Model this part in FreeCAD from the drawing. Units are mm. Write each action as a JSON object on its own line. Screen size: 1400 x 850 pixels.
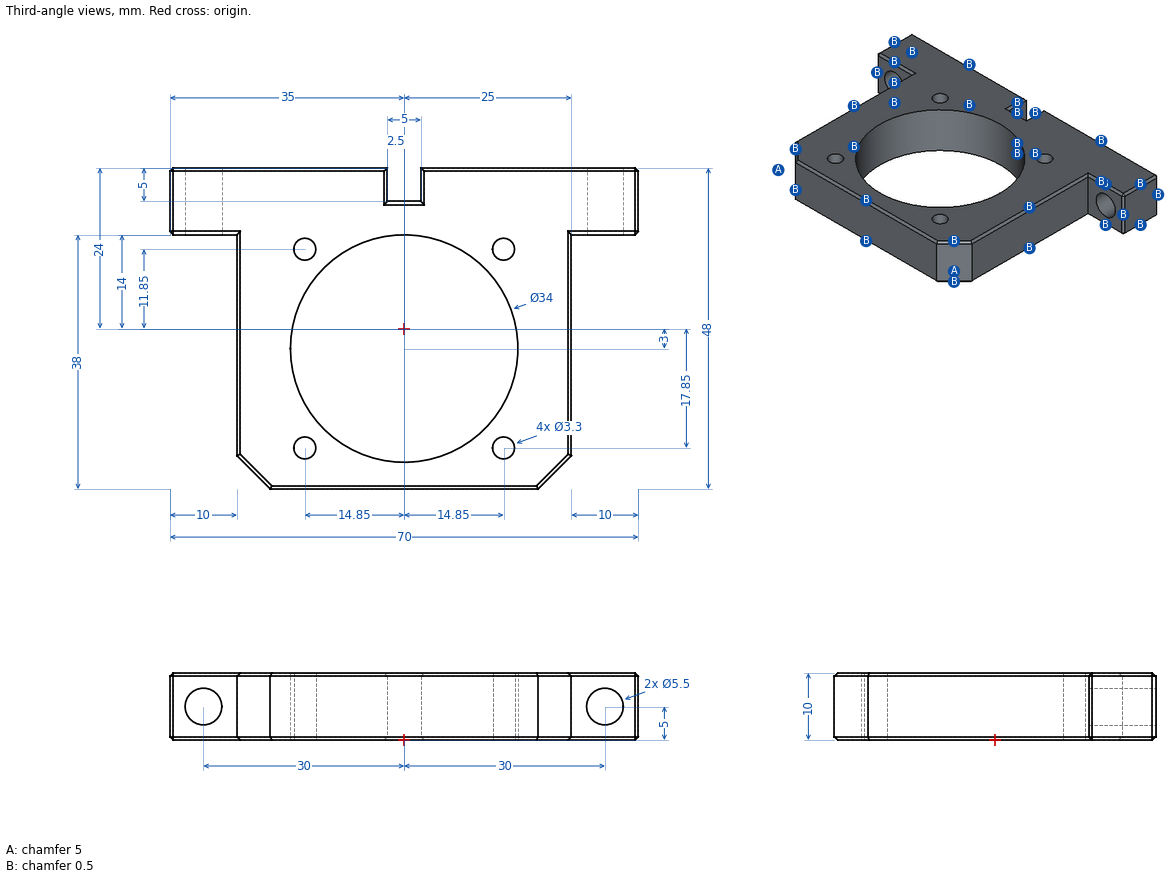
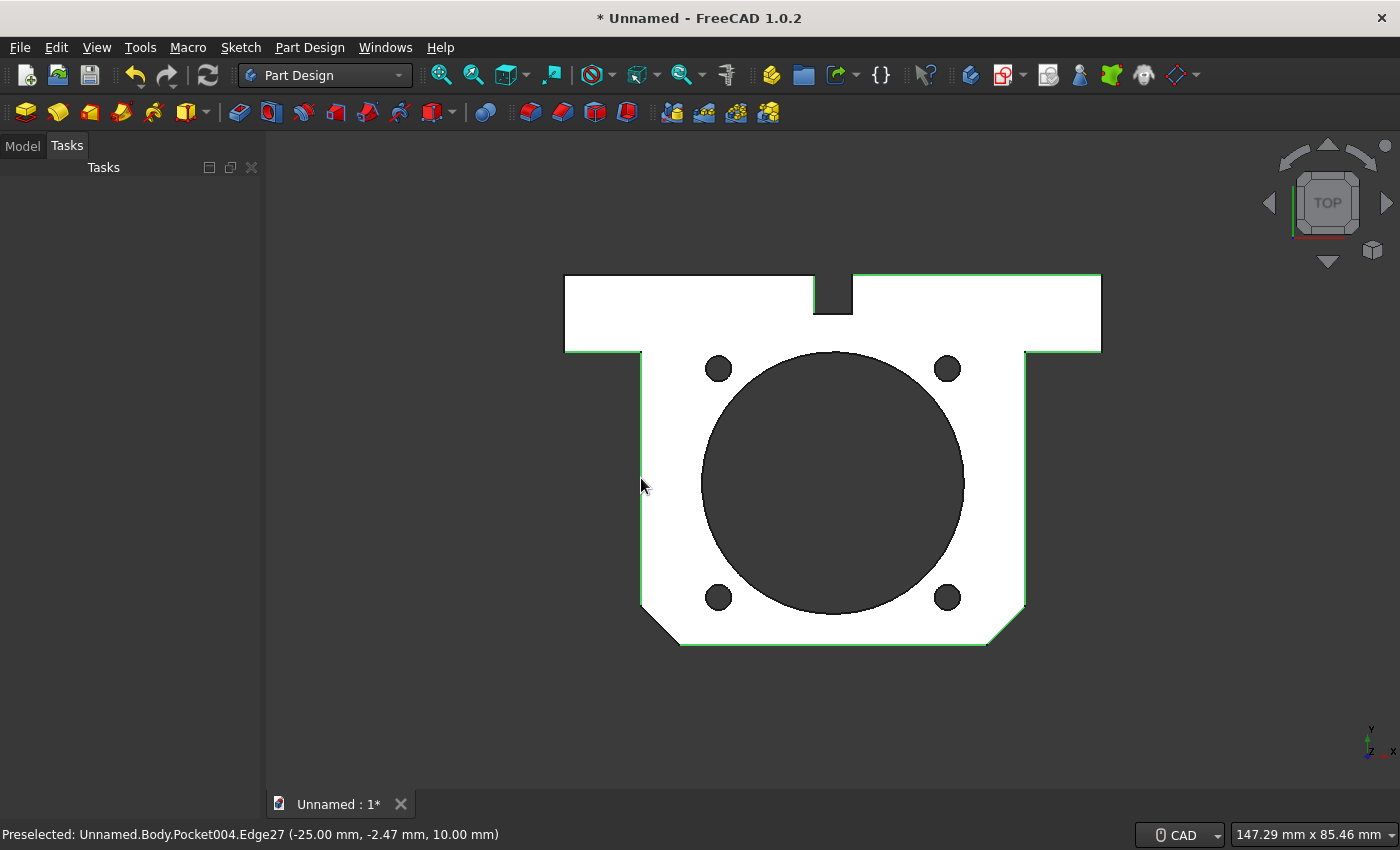
{"action": "left_click", "coordinate": [660, 625], "text": "ctrl"}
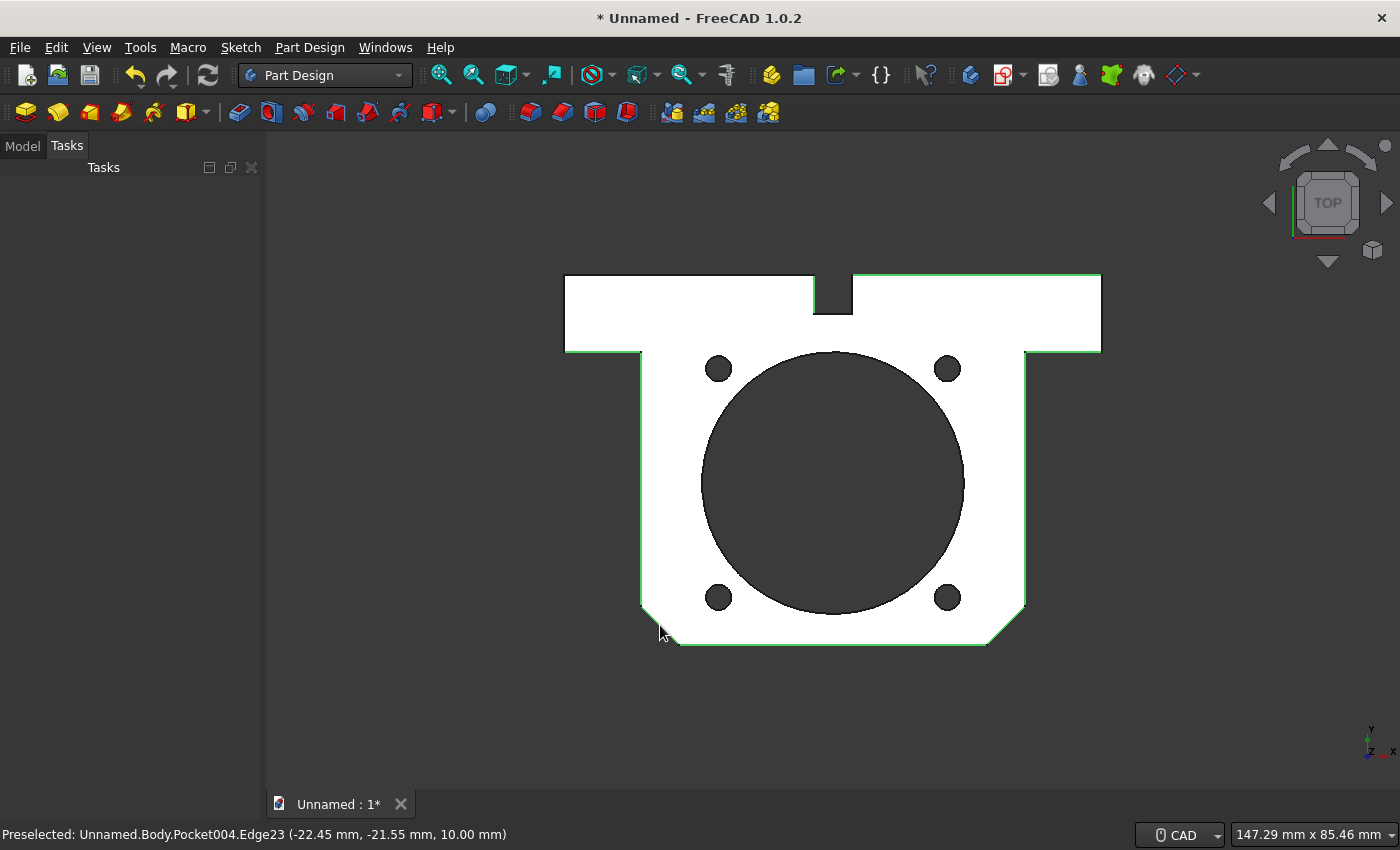
{"action": "left_click", "coordinate": [689, 274], "text": "ctrl"}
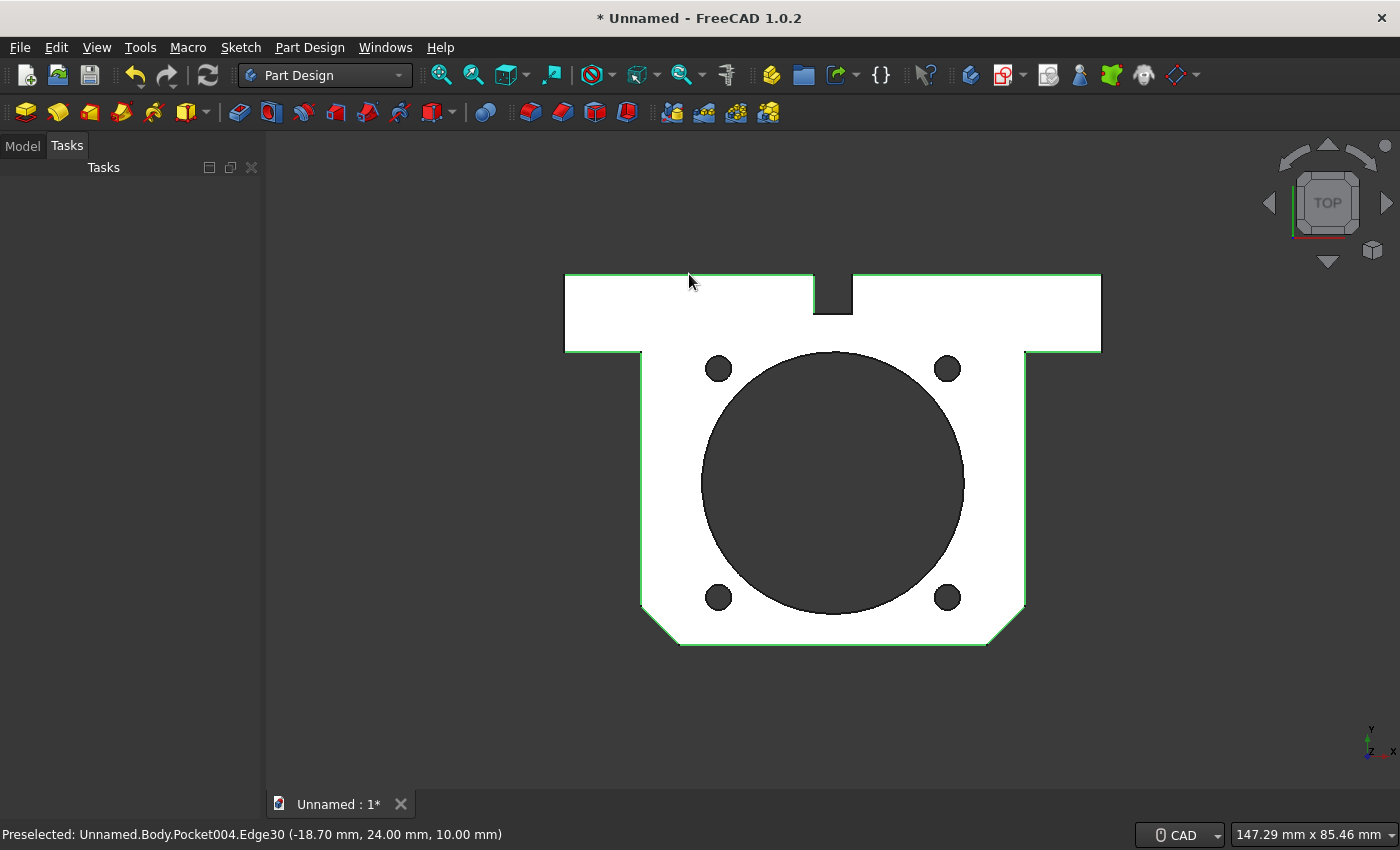
{"action": "left_click", "coordinate": [833, 313], "text": "ctrl"}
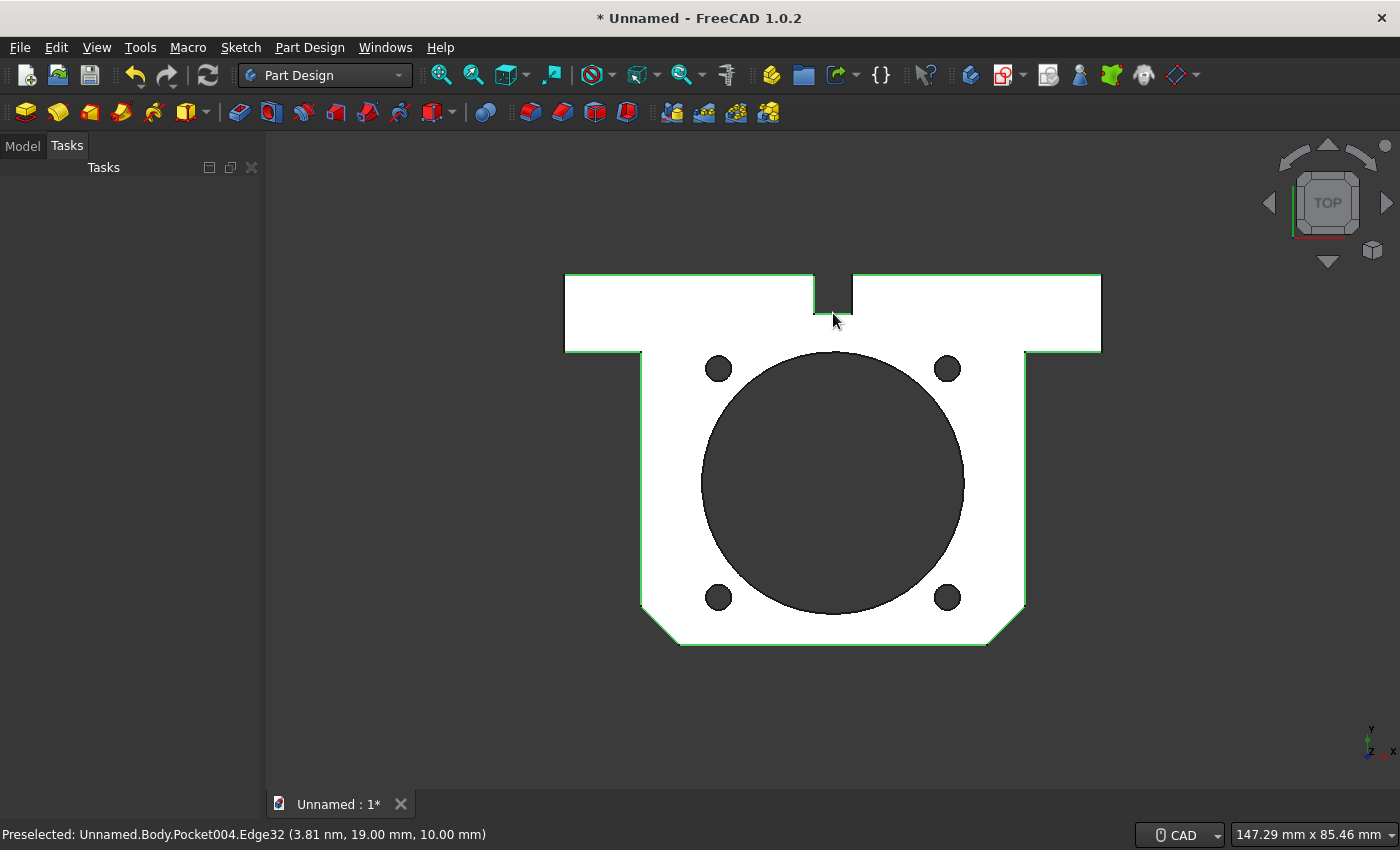
{"action": "left_click", "coordinate": [852, 293], "text": "ctrl"}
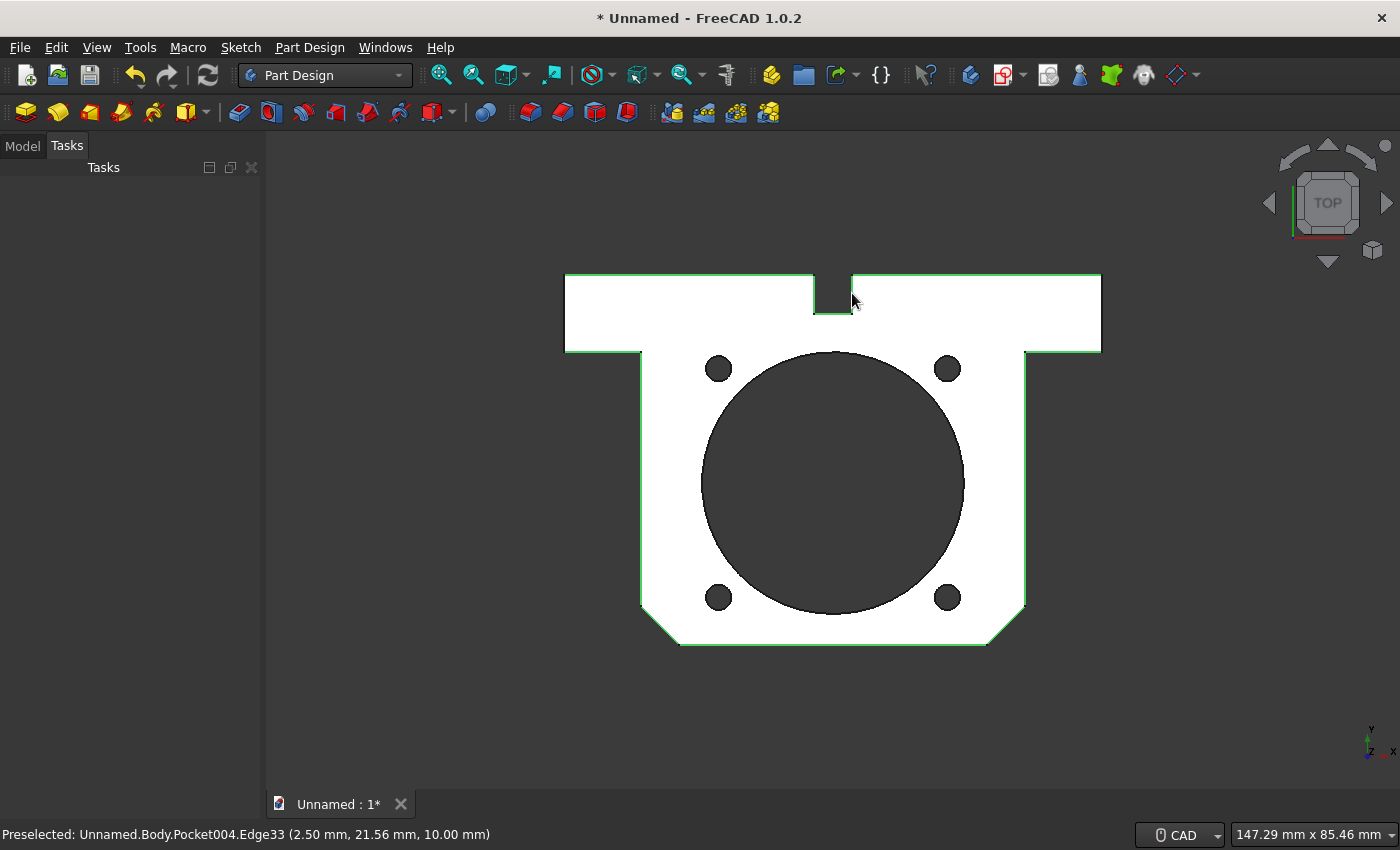
{"action": "key", "text": "0"}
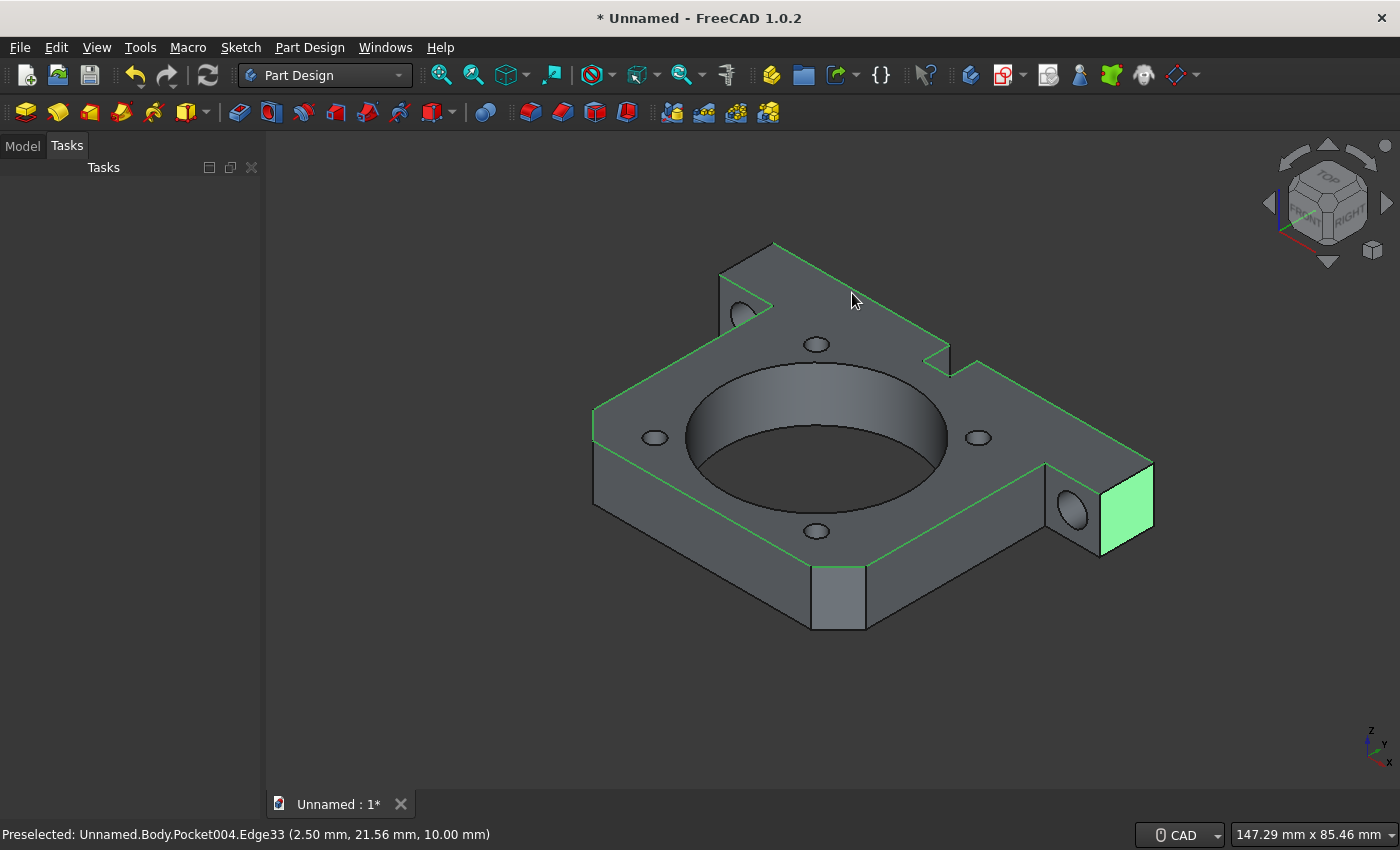
{"action": "key", "text": "1"}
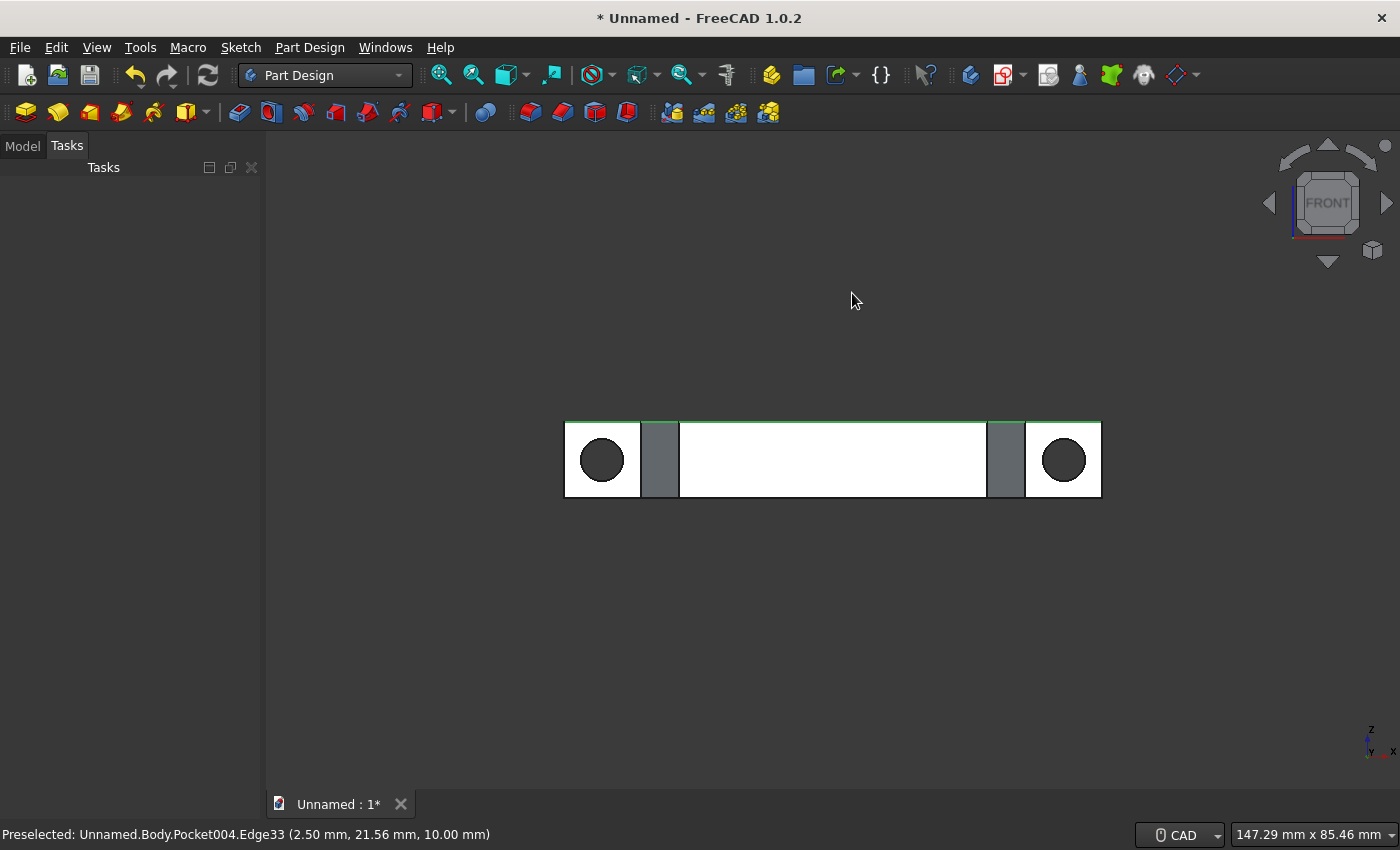
{"action": "left_click", "coordinate": [602, 497], "text": "ctrl"}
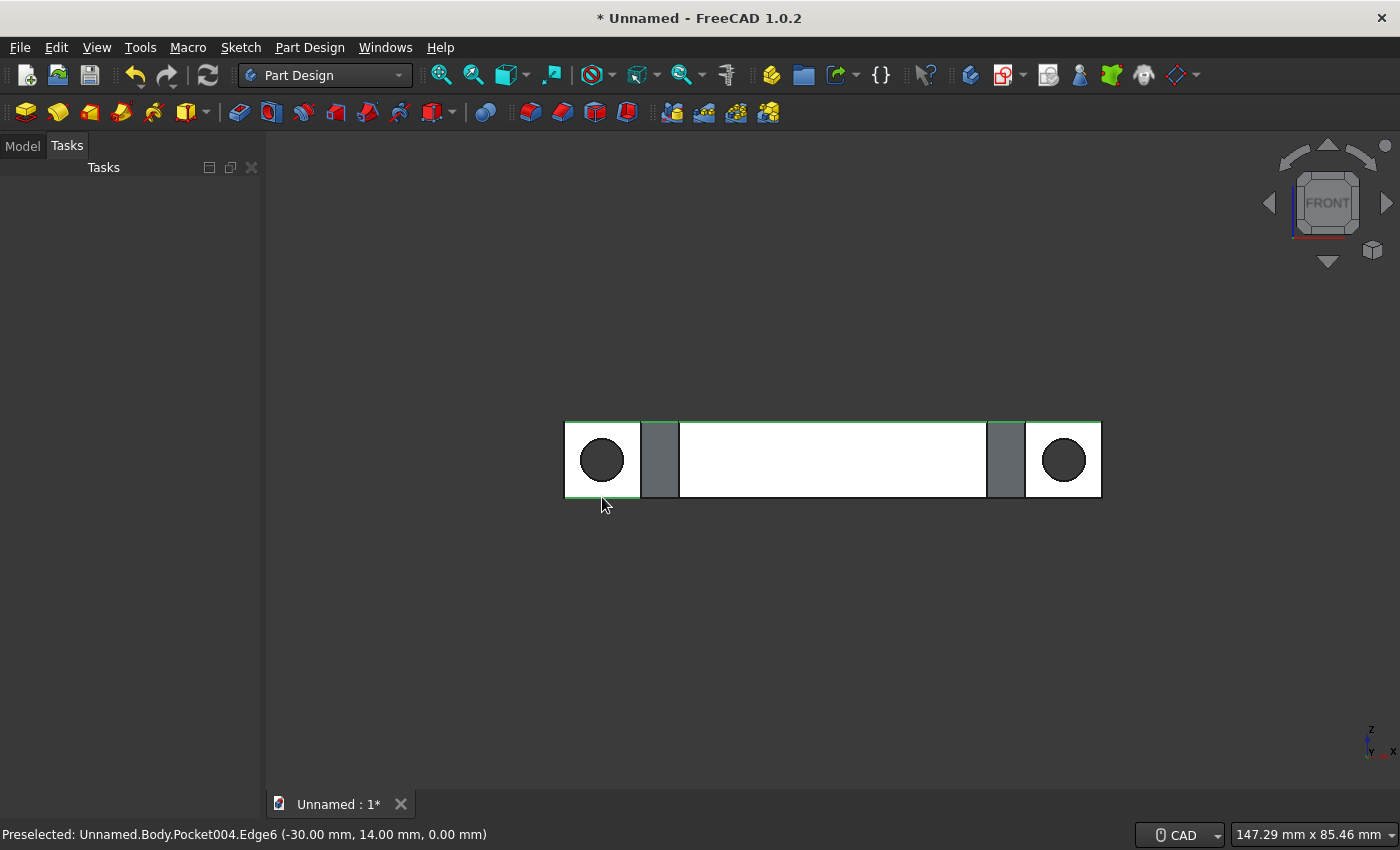
{"action": "left_click", "coordinate": [1064, 497], "text": "ctrl"}